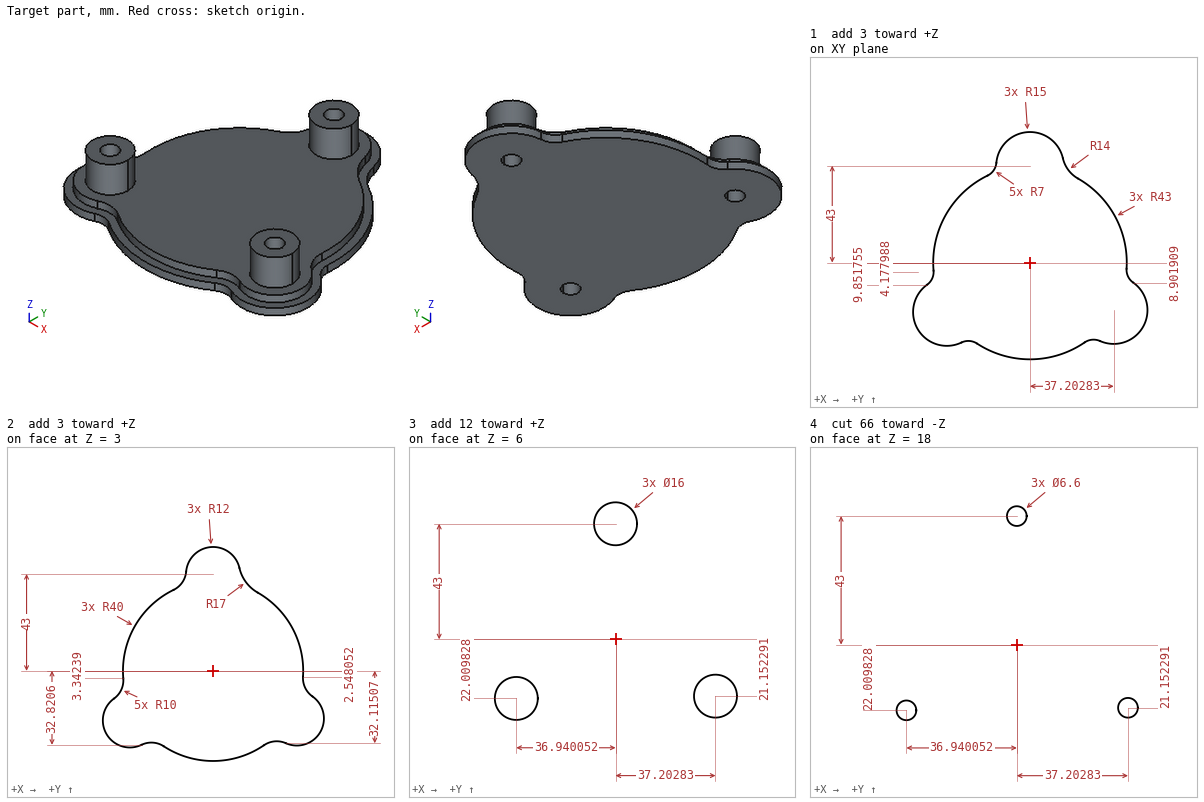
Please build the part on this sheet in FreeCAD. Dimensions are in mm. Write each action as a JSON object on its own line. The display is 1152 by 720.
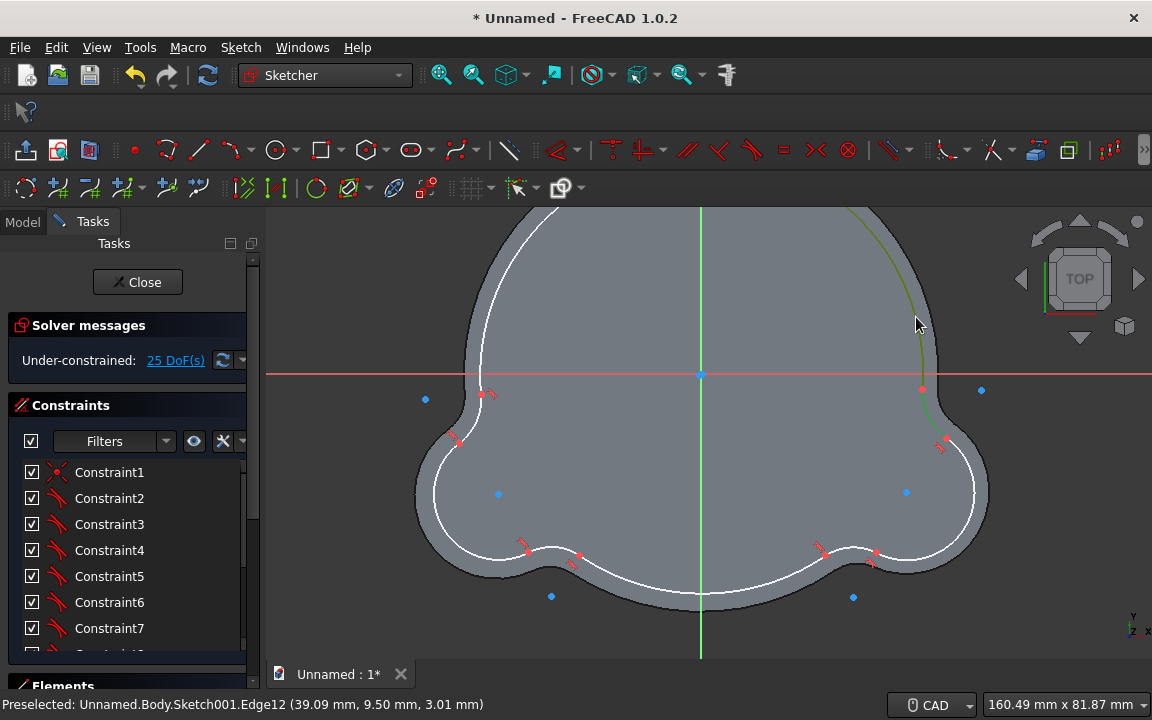
{"action": "left_click", "coordinate": [752, 150]}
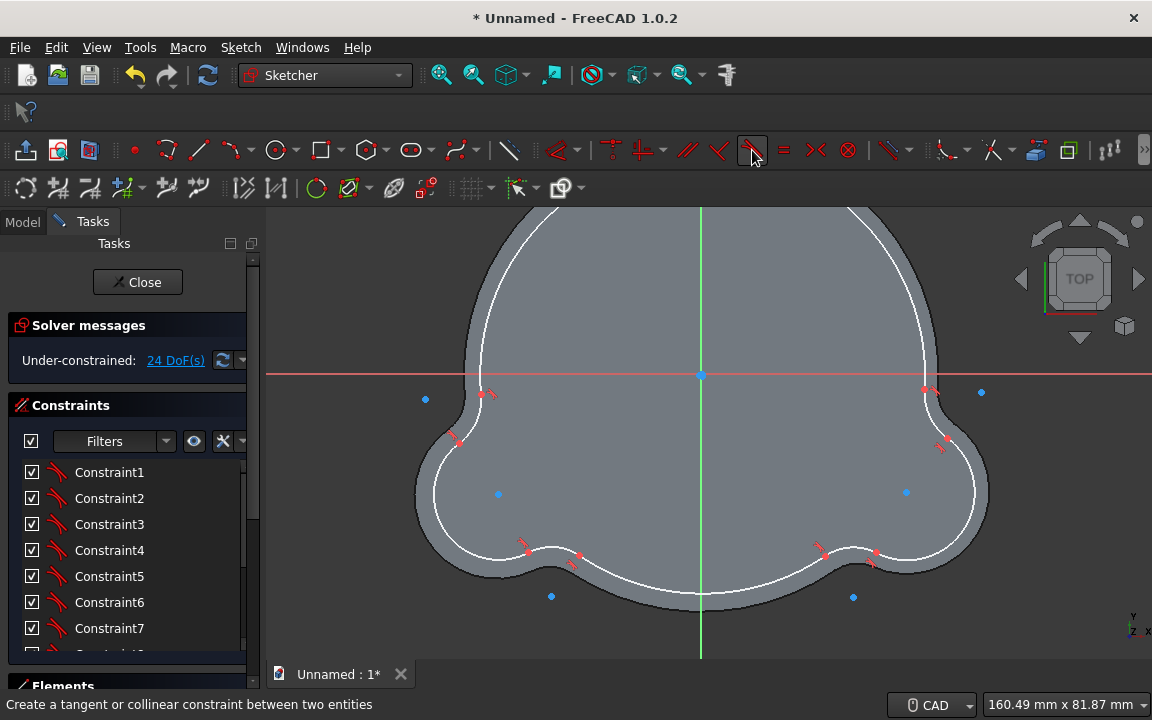
{"action": "left_click", "coordinate": [489, 316]}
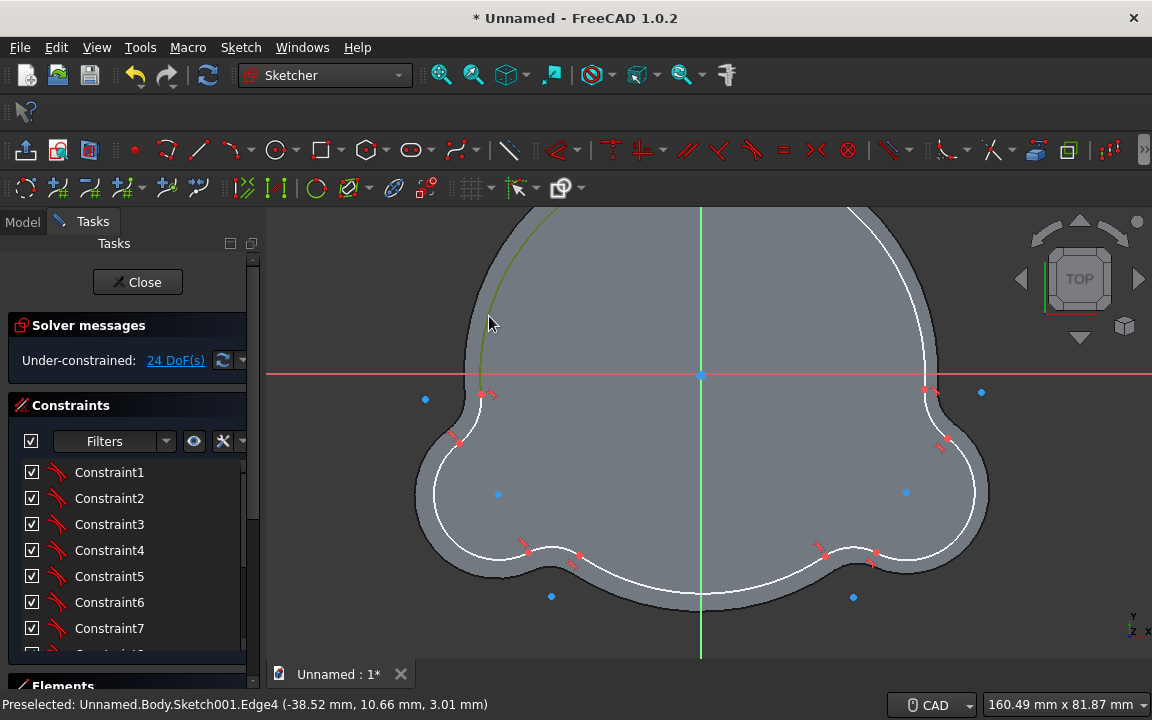
{"action": "left_click", "coordinate": [651, 587]}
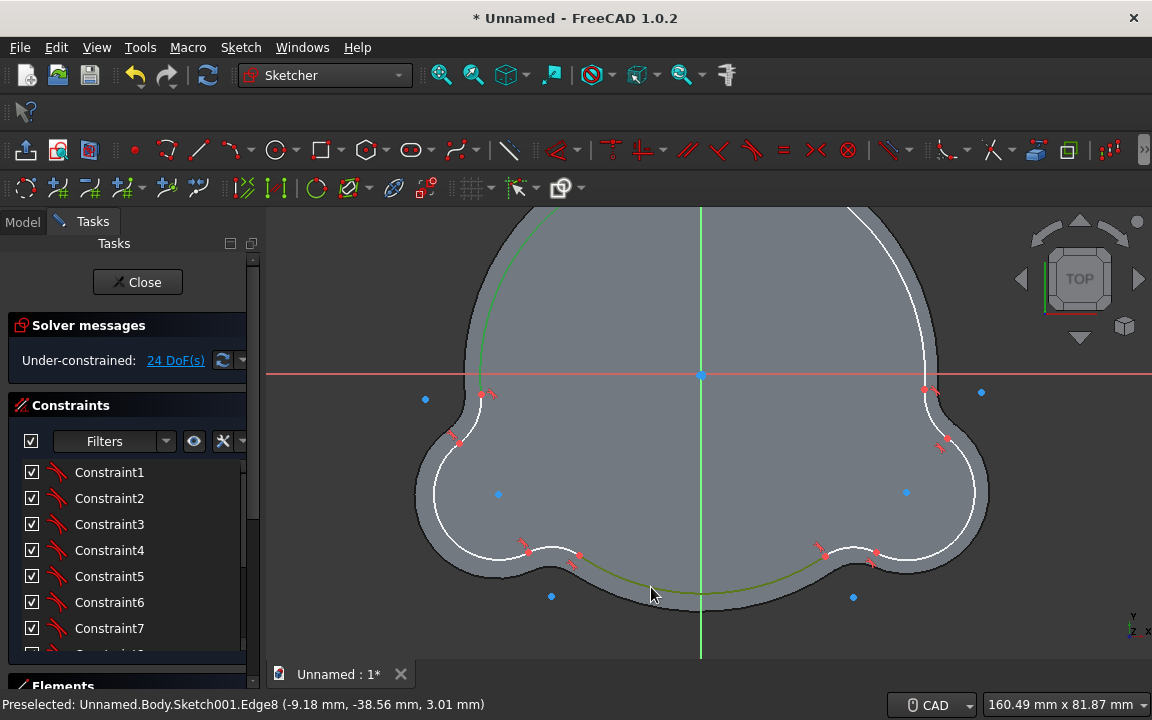
{"action": "left_click", "coordinate": [612, 150]}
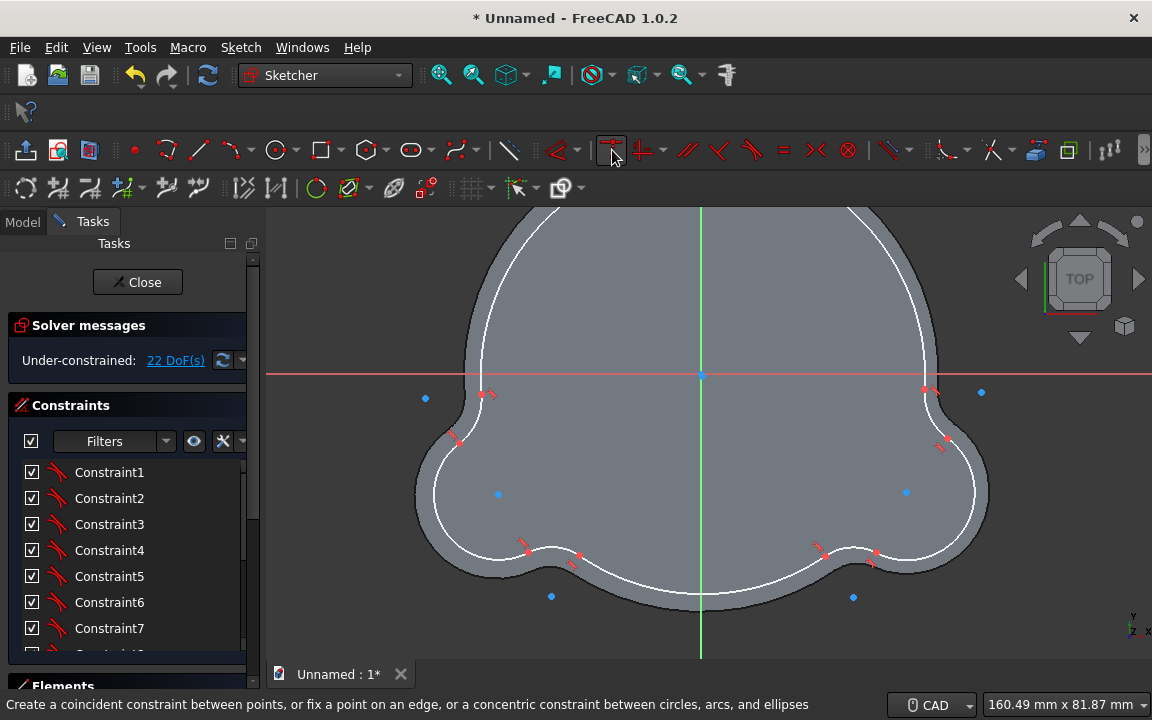
{"action": "left_click", "coordinate": [489, 316]}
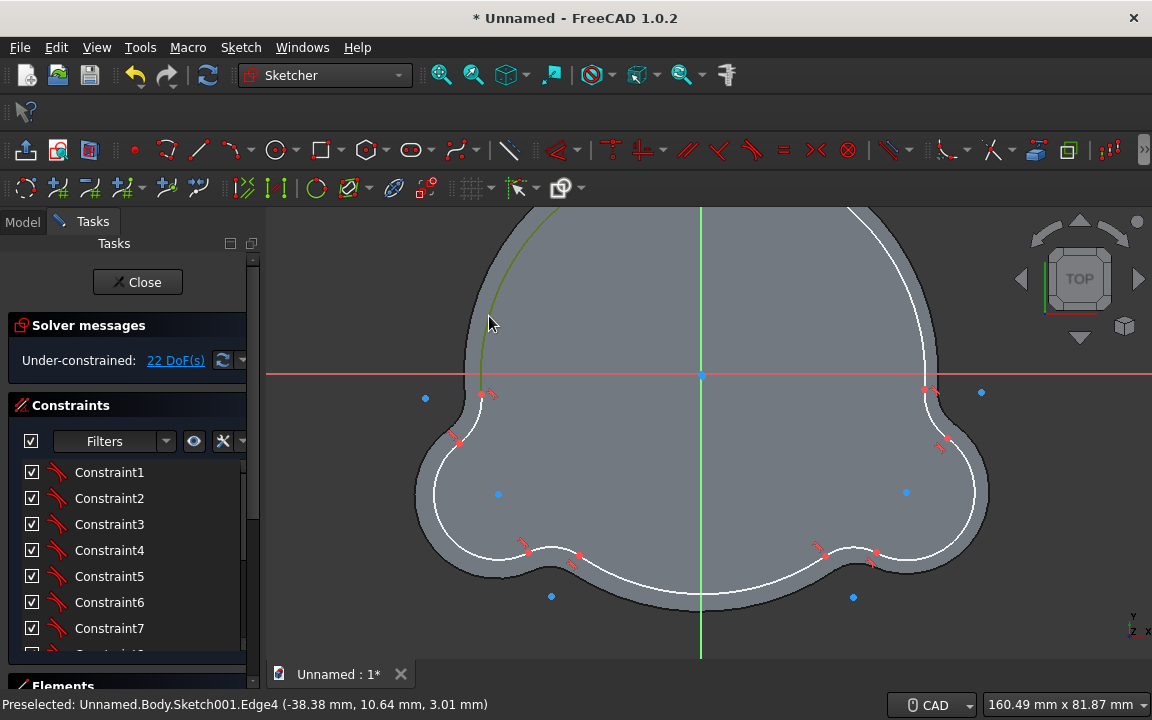
{"action": "left_click", "coordinate": [917, 317]}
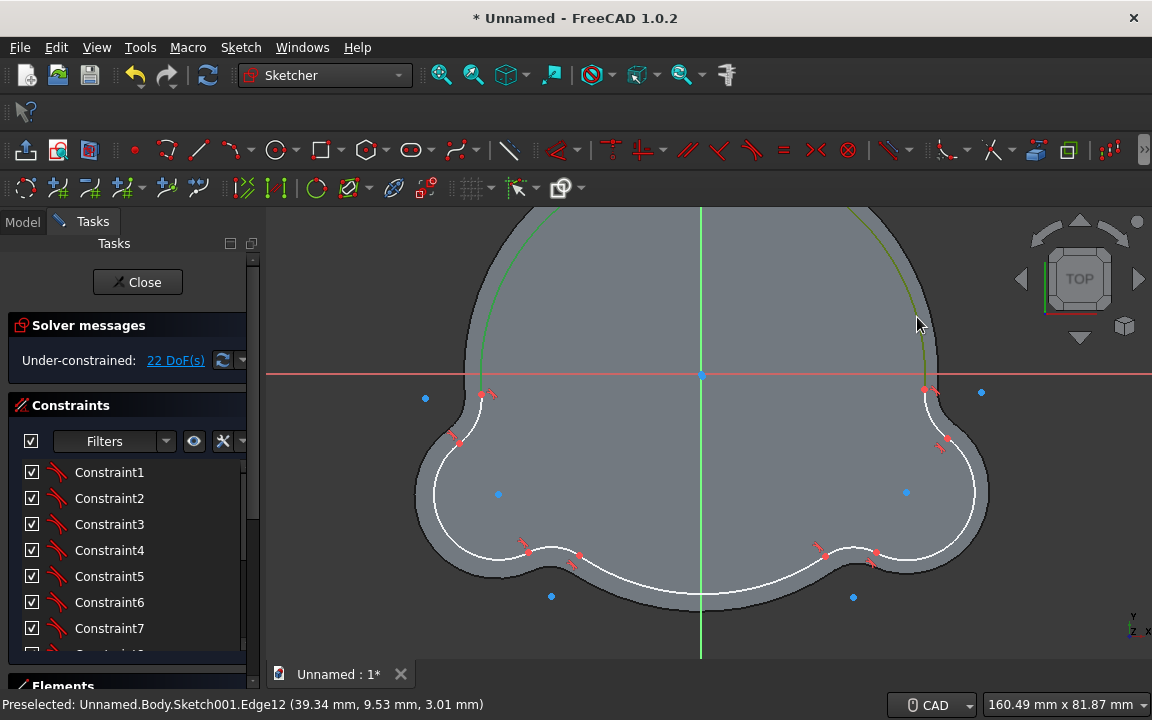
{"action": "left_click", "coordinate": [612, 150]}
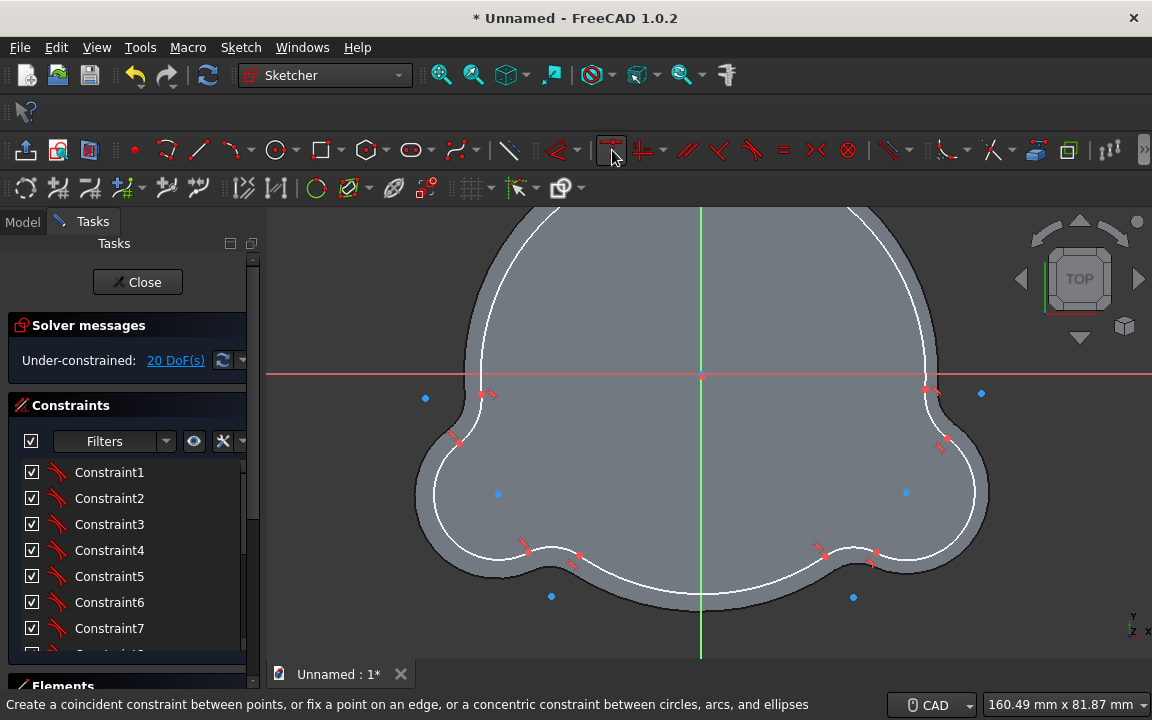
{"action": "left_click_drag", "start_coordinate": [691, 364], "coordinate": [713, 387]}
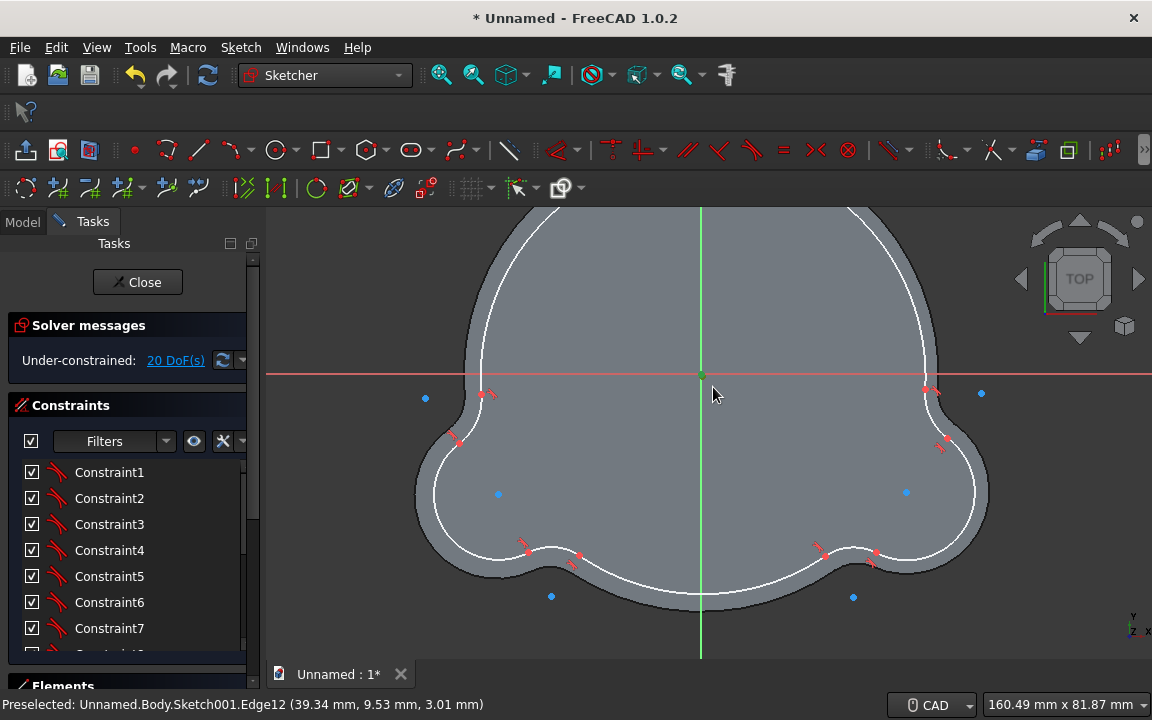
{"action": "left_click", "coordinate": [612, 150]}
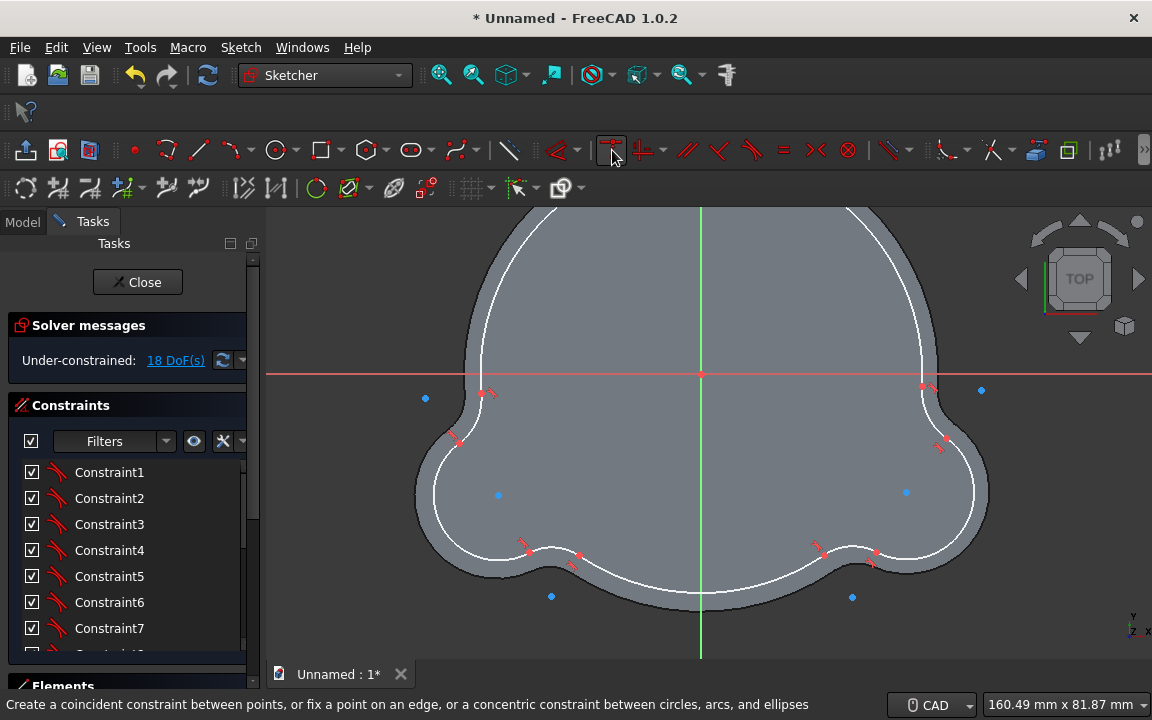
{"action": "scroll", "coordinate": [565, 554], "scroll_direction": "down", "scroll_amount": 3}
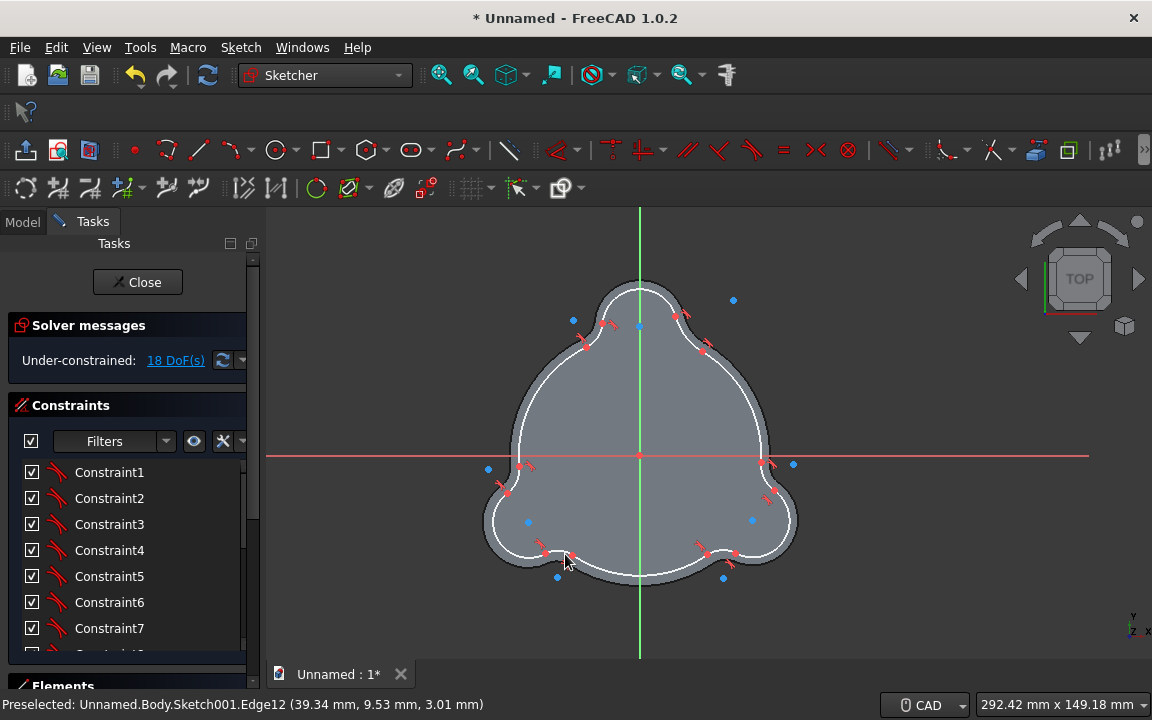
{"action": "scroll", "coordinate": [594, 342], "scroll_direction": "up", "scroll_amount": 3}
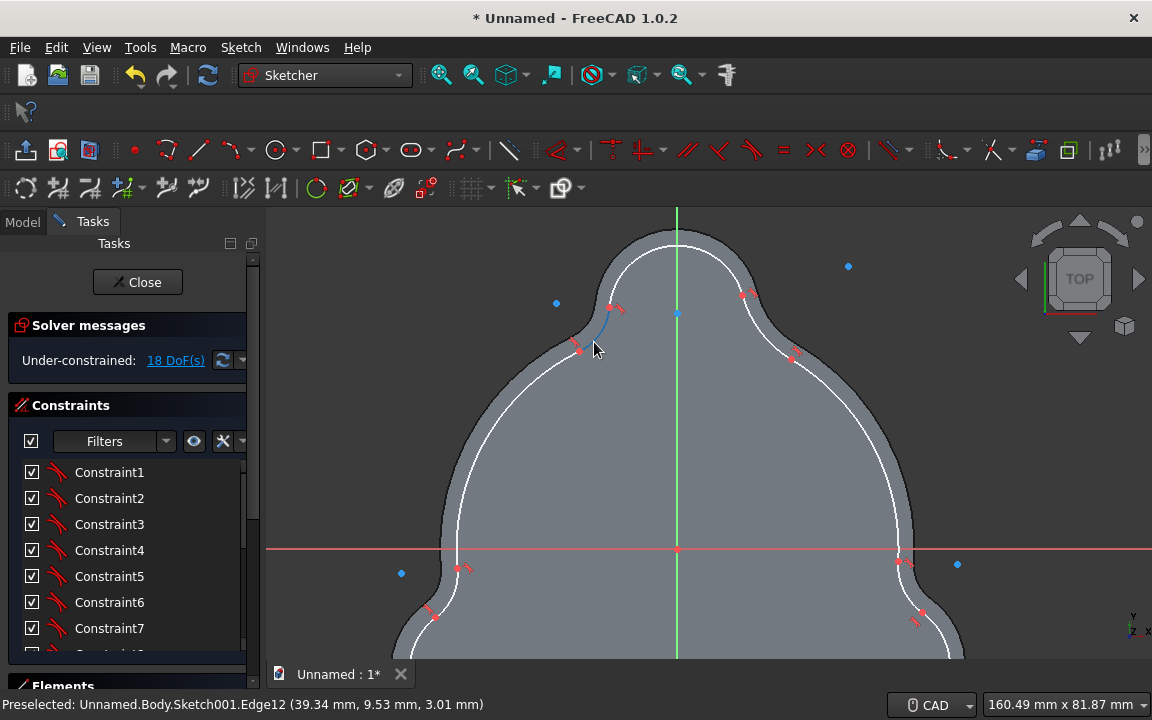
{"action": "left_click", "coordinate": [593, 342]}